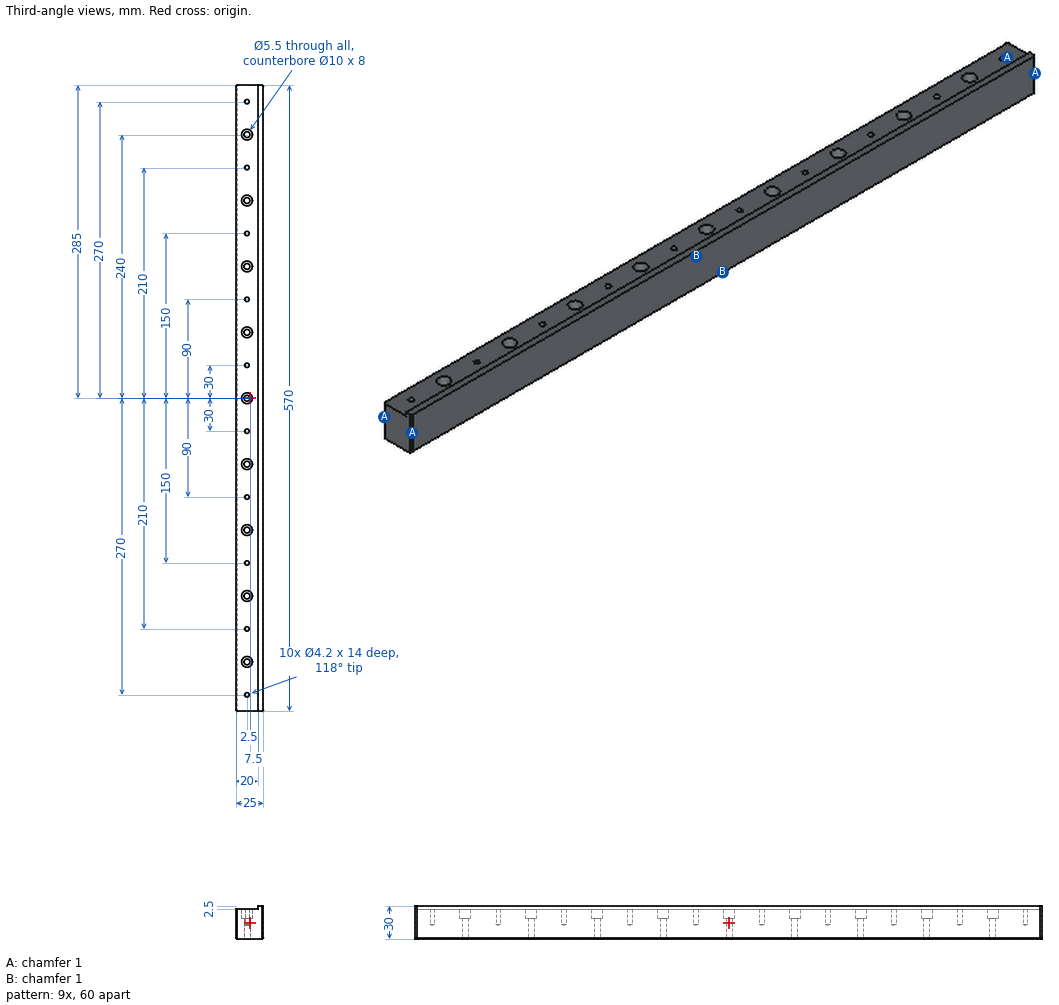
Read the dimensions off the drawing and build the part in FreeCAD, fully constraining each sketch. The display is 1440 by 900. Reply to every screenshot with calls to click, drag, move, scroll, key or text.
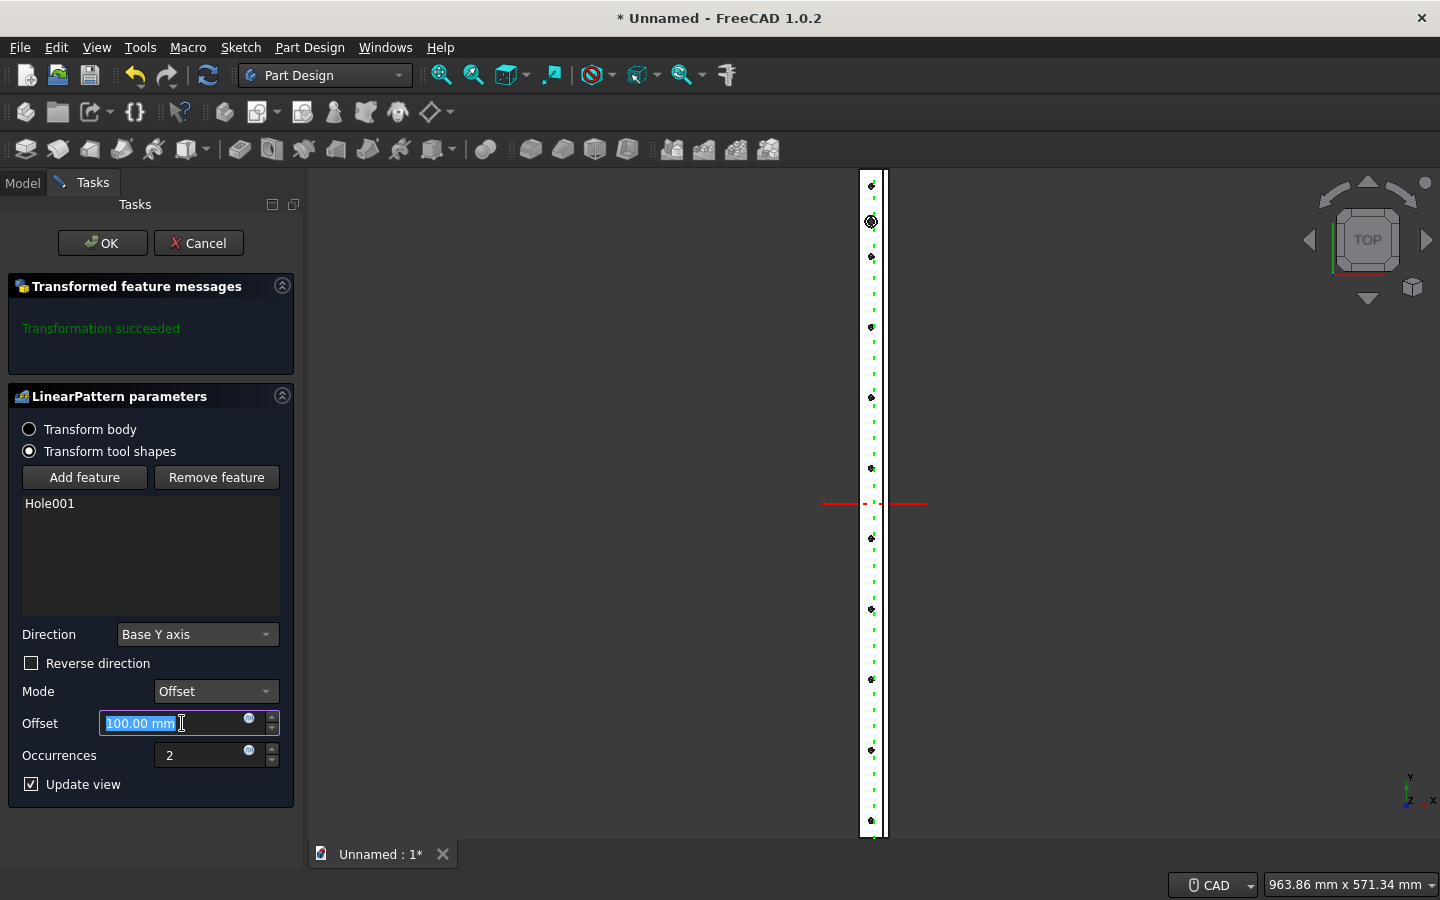
text(60)
key(Tab)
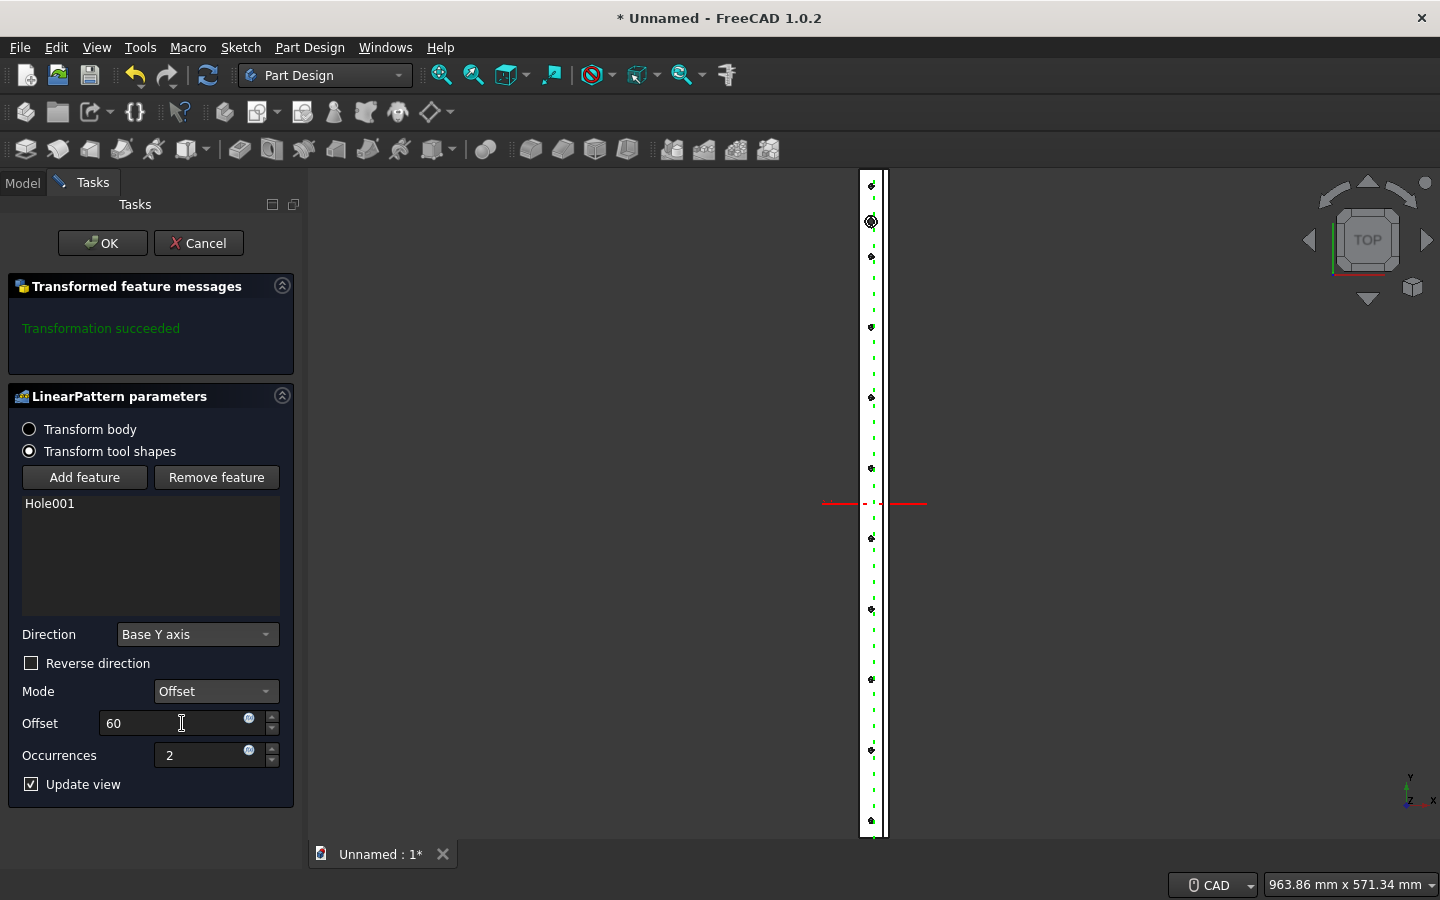
triple_click(209, 755)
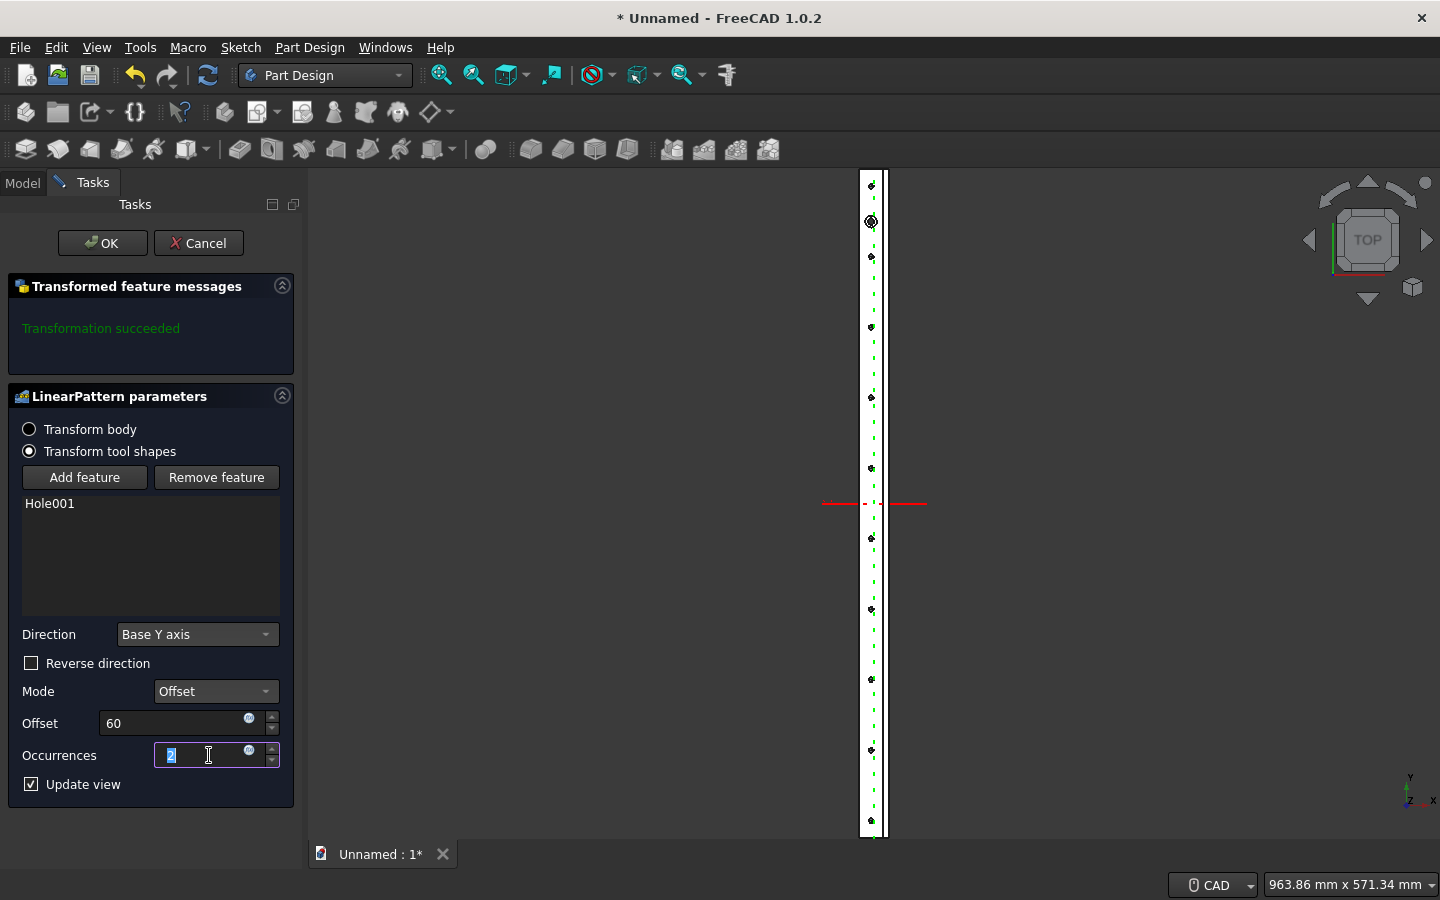
text(9)
key(Tab)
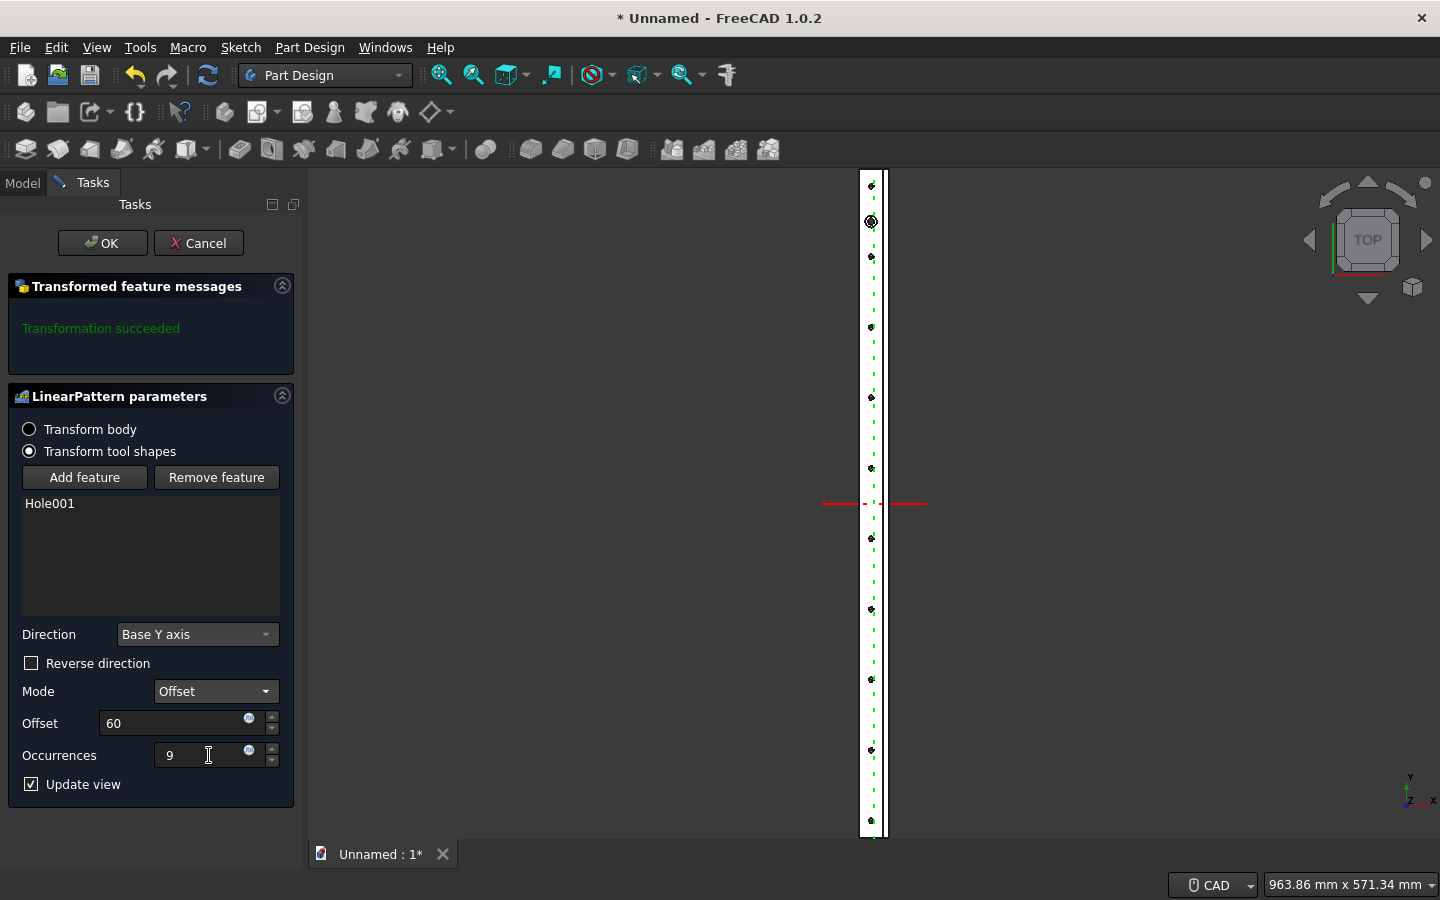
click(30, 663)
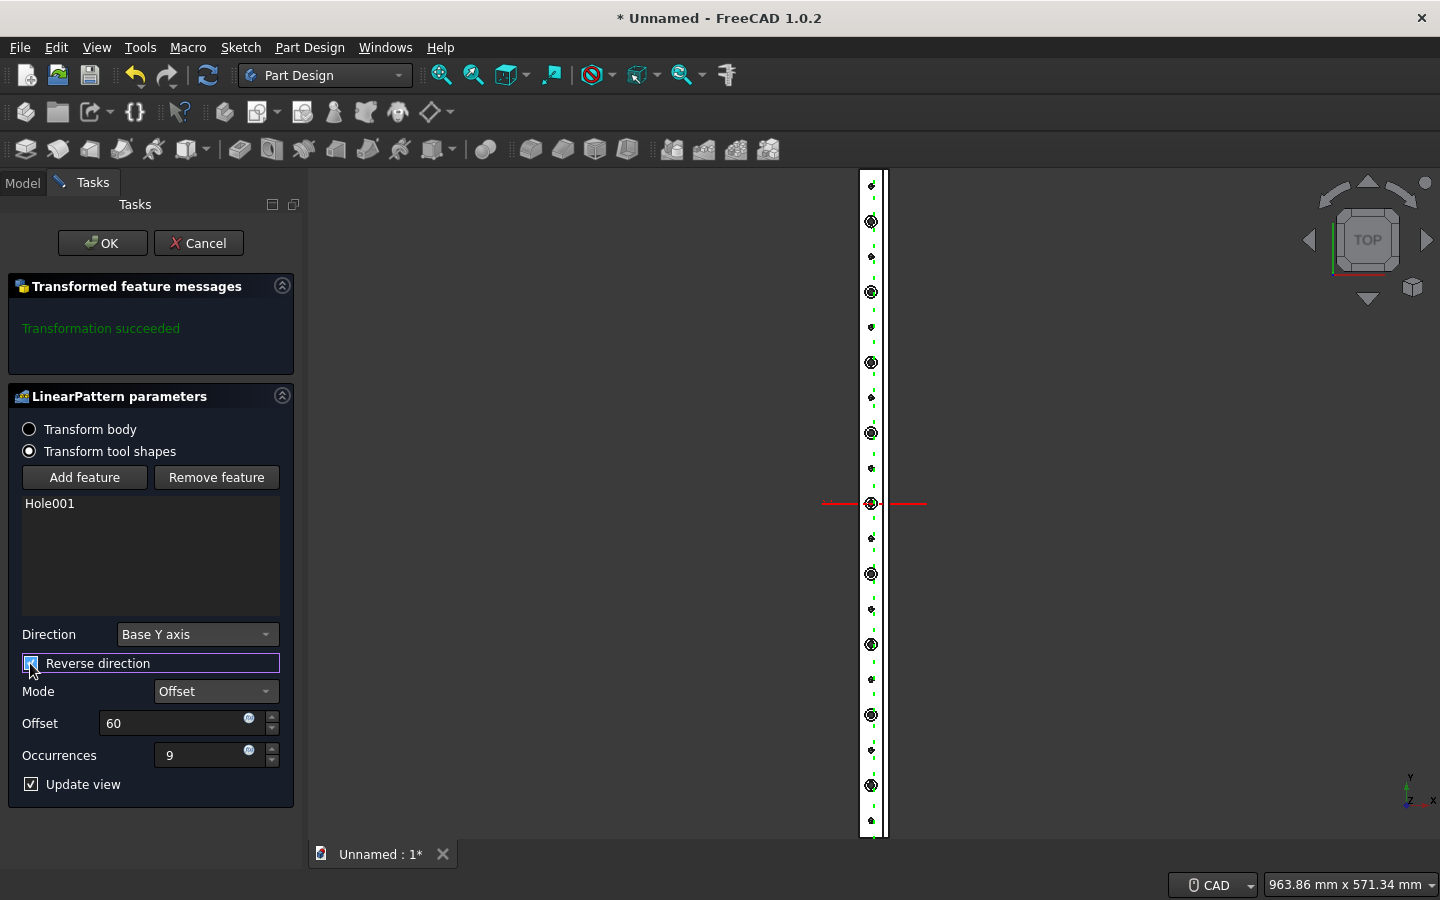
click(103, 243)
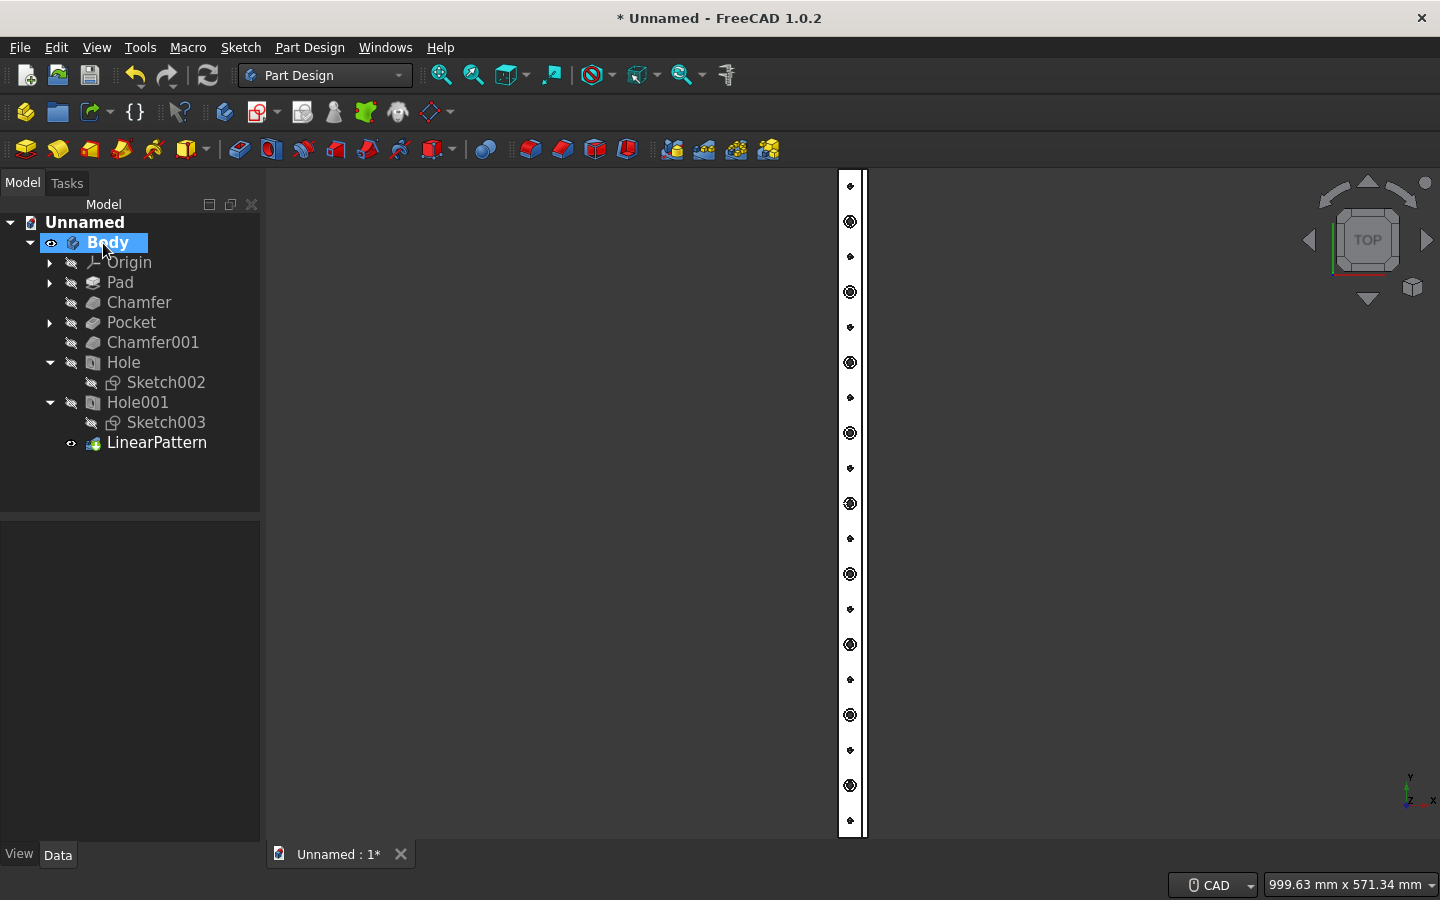
key(0)